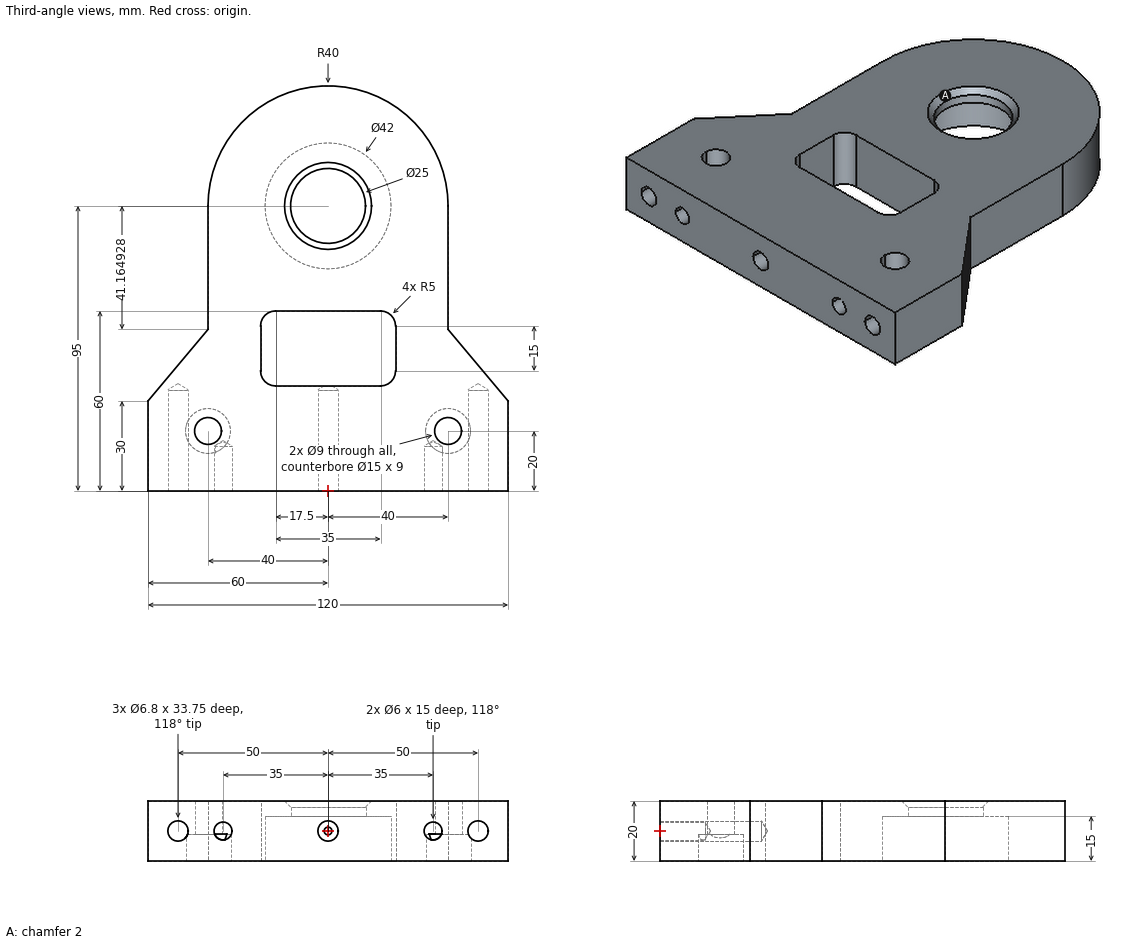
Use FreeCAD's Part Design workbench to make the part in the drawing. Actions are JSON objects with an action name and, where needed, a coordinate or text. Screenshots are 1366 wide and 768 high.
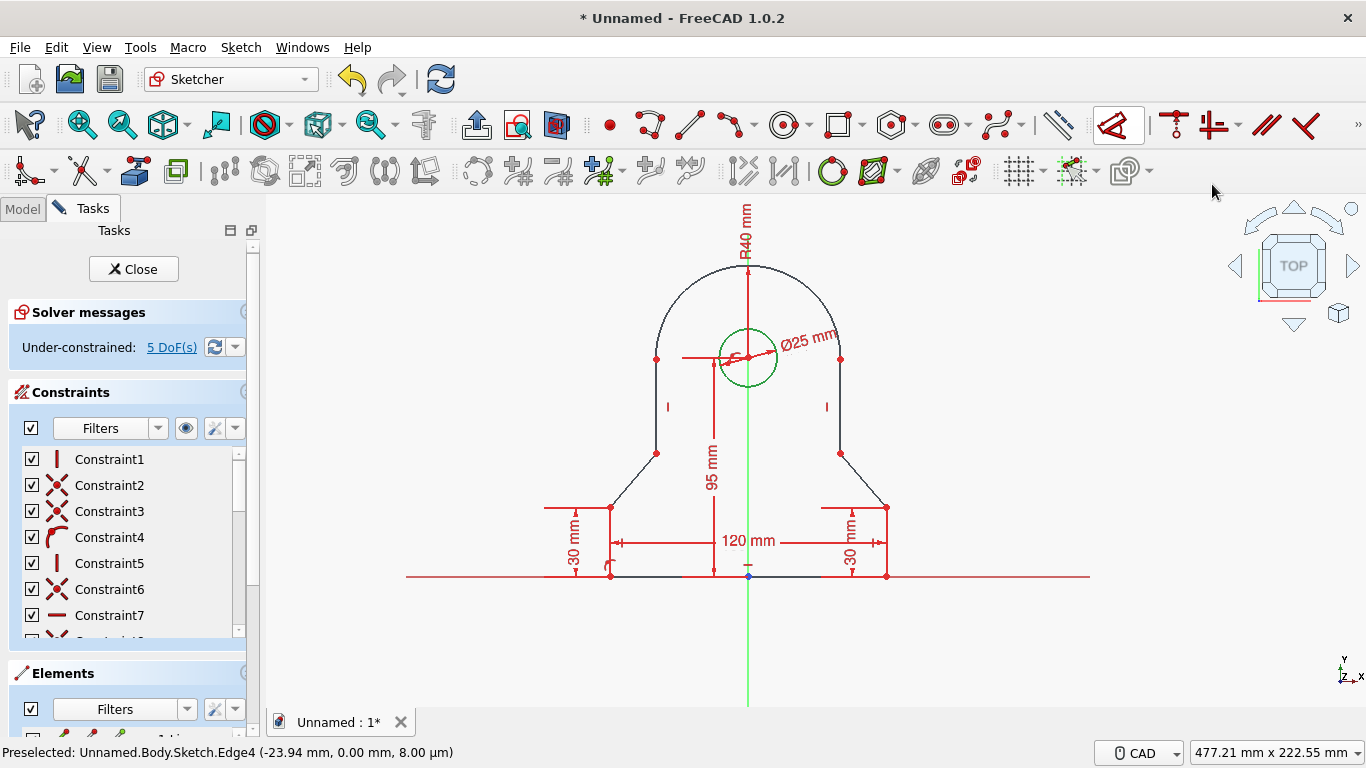
{"action": "left_click", "coordinate": [656, 359]}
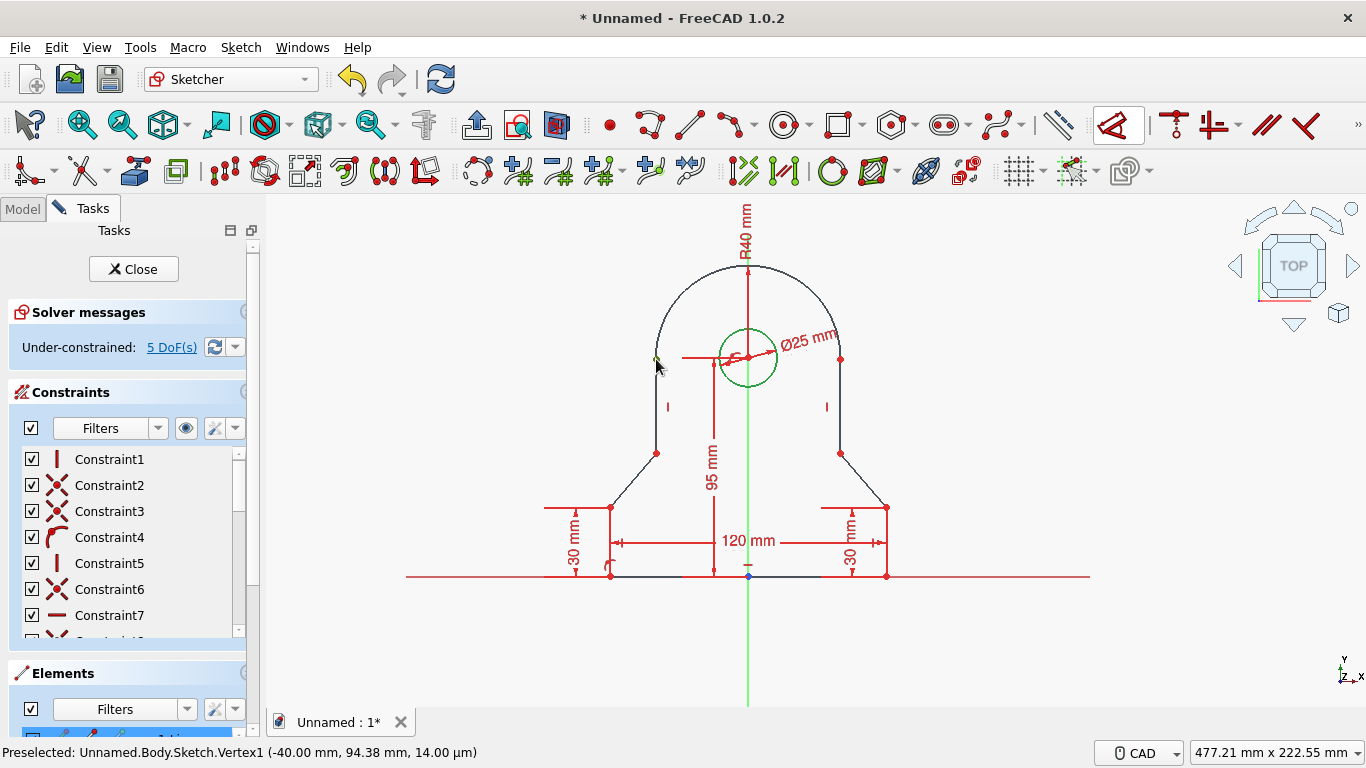
{"action": "key", "text": "i"}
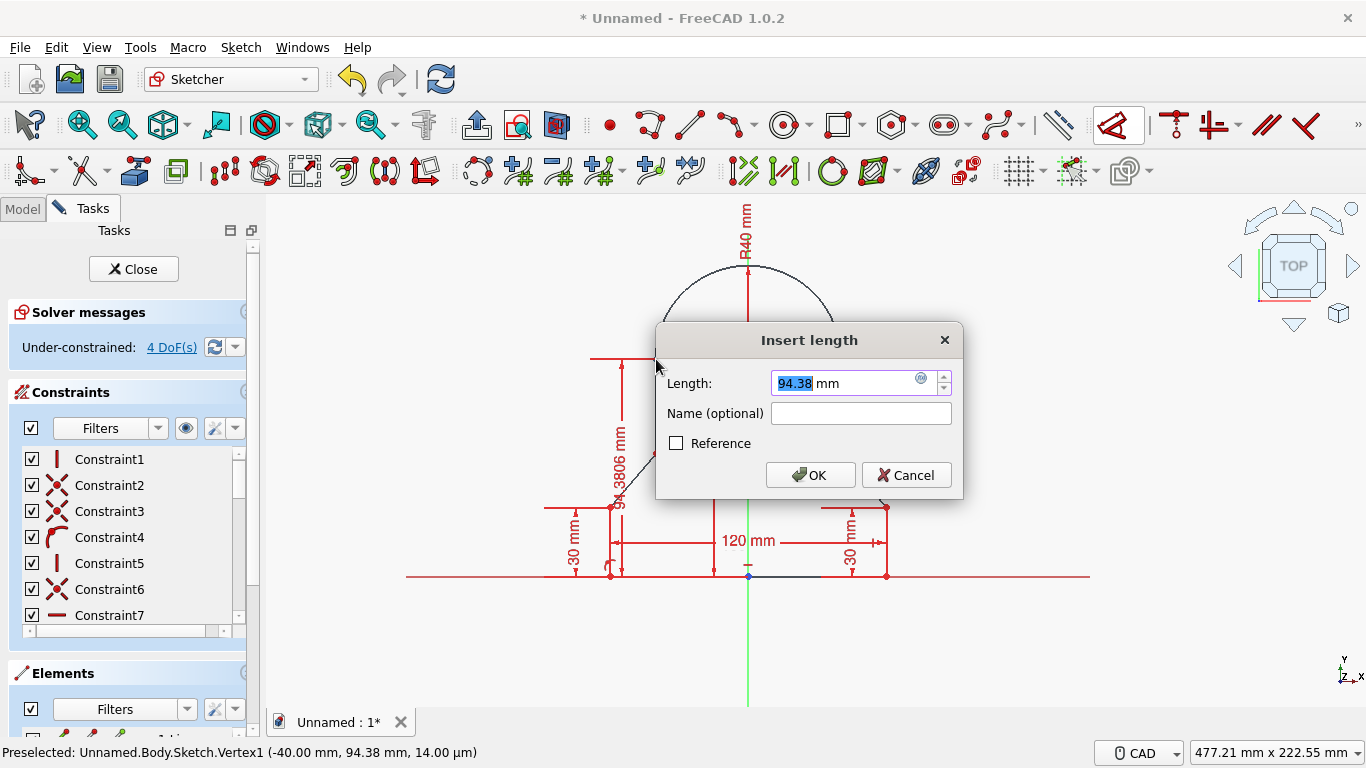
{"action": "type", "text": "95"}
{"action": "key", "text": "Return"}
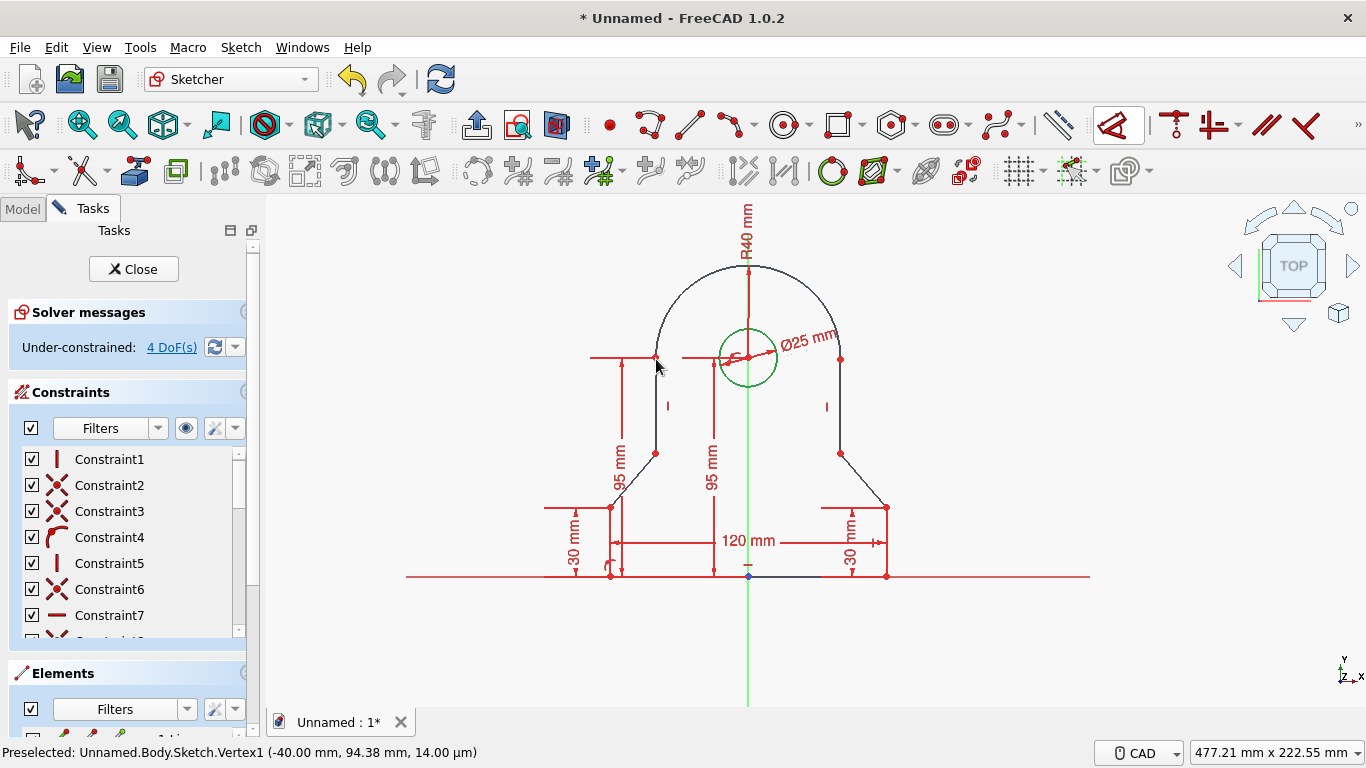
{"action": "left_click", "coordinate": [610, 508]}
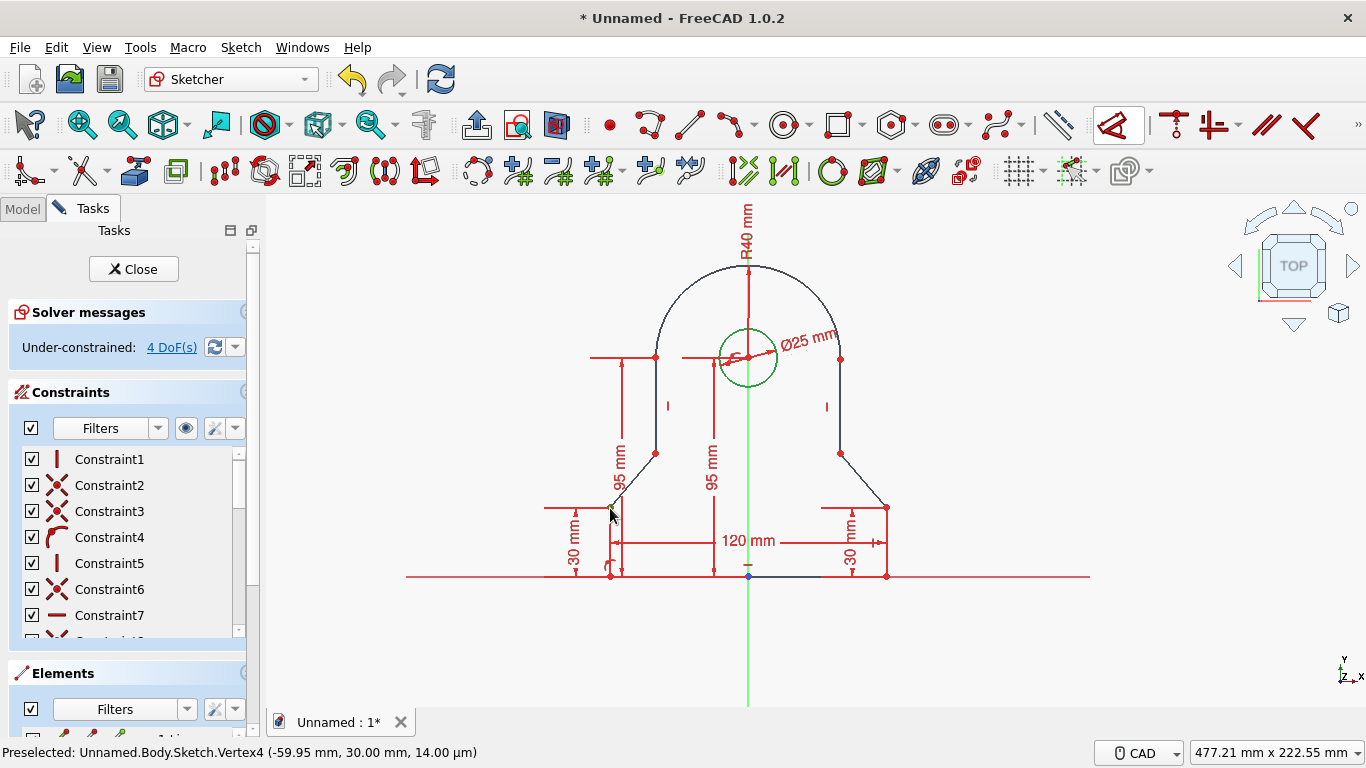
{"action": "left_click", "coordinate": [1138, 126]}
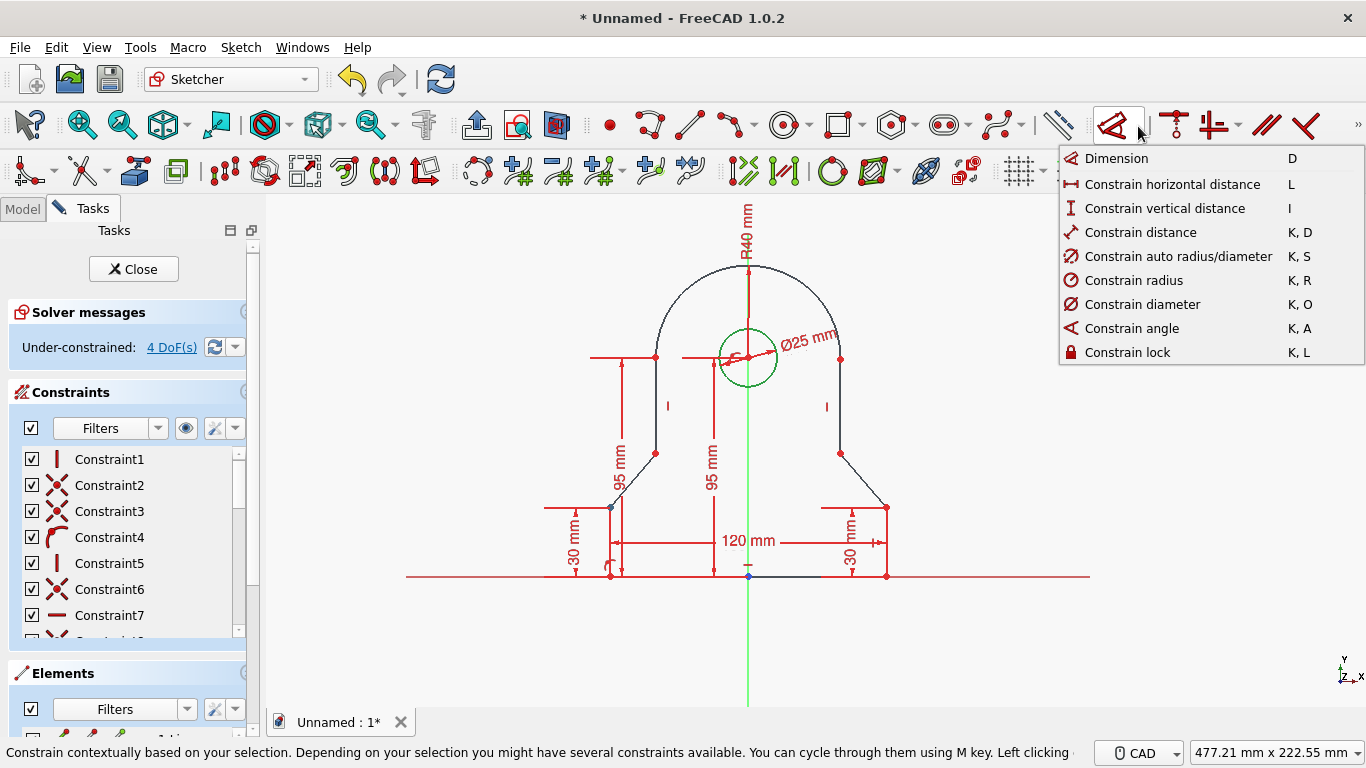
{"action": "left_click", "coordinate": [1212, 184]}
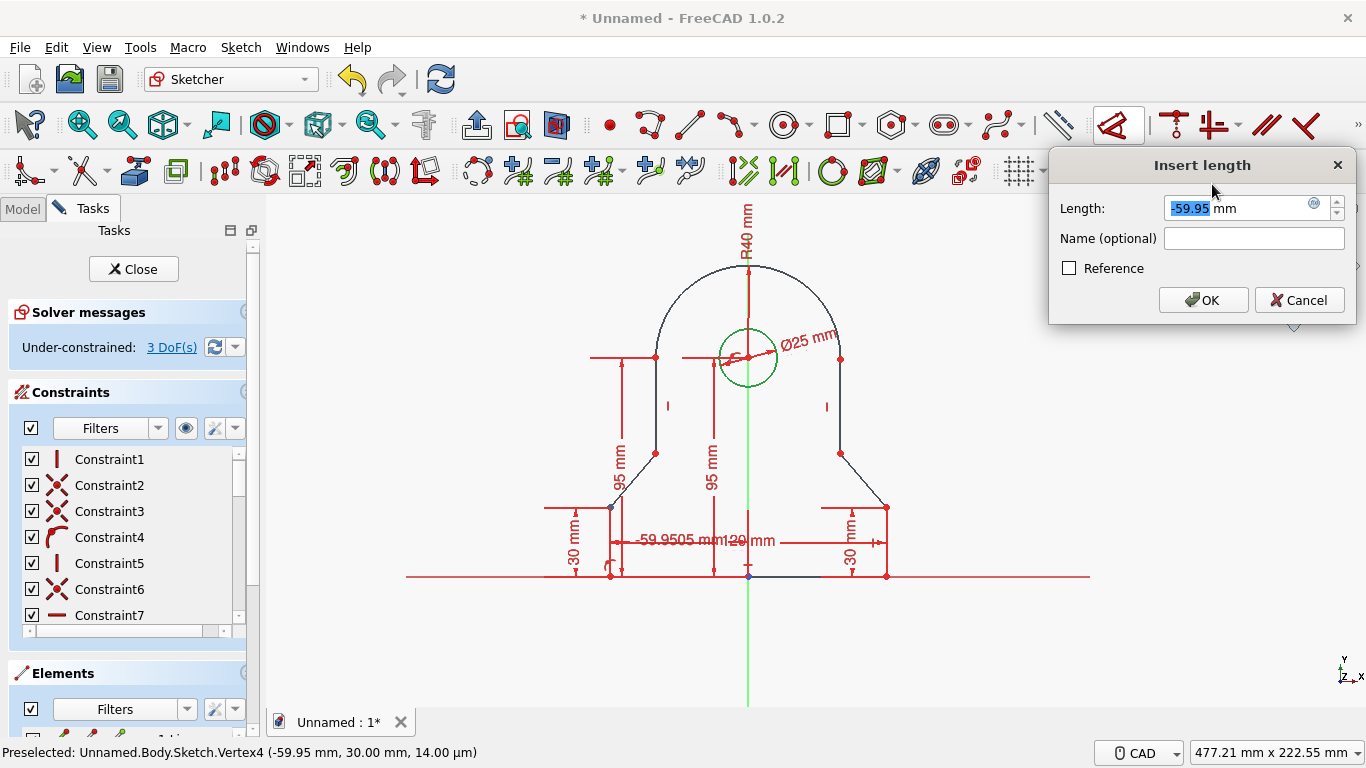
{"action": "type", "text": "-60"}
{"action": "key", "text": "Return"}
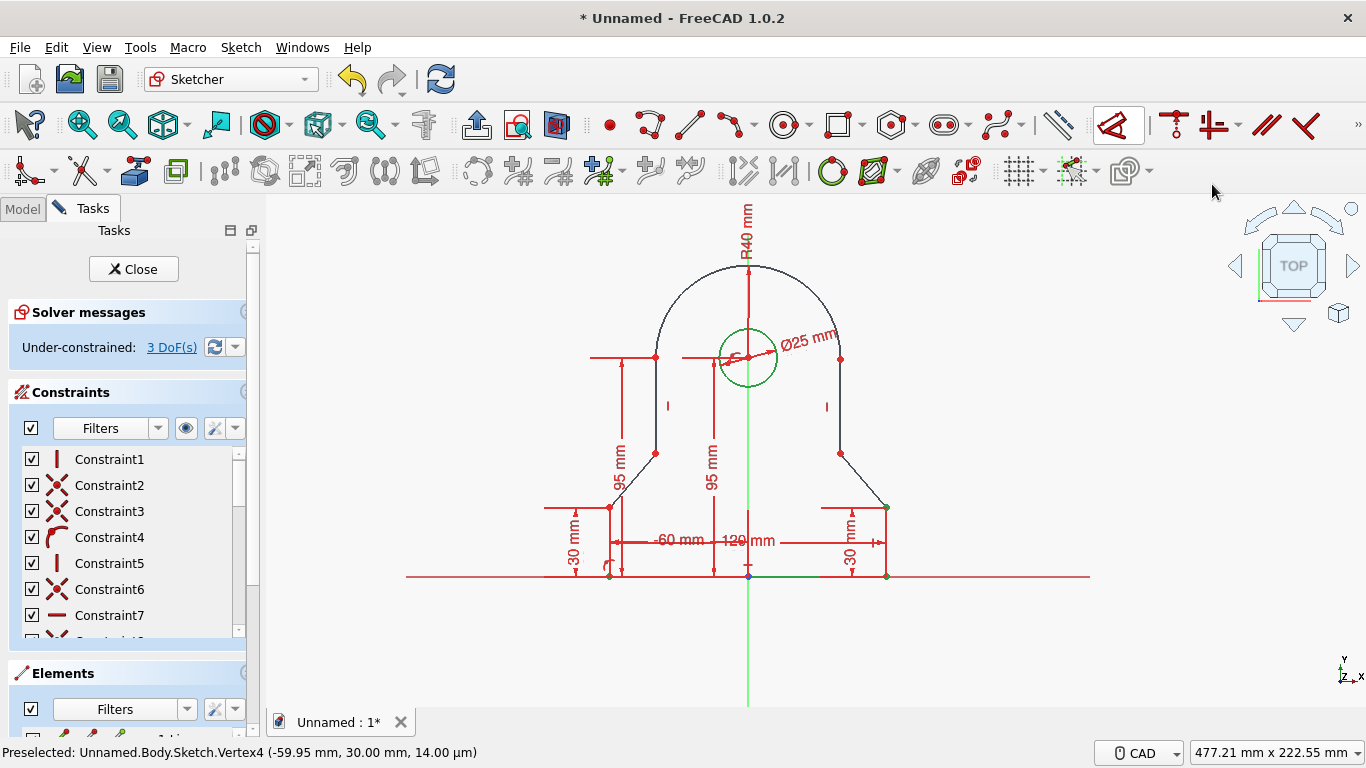
{"action": "left_click", "coordinate": [840, 359]}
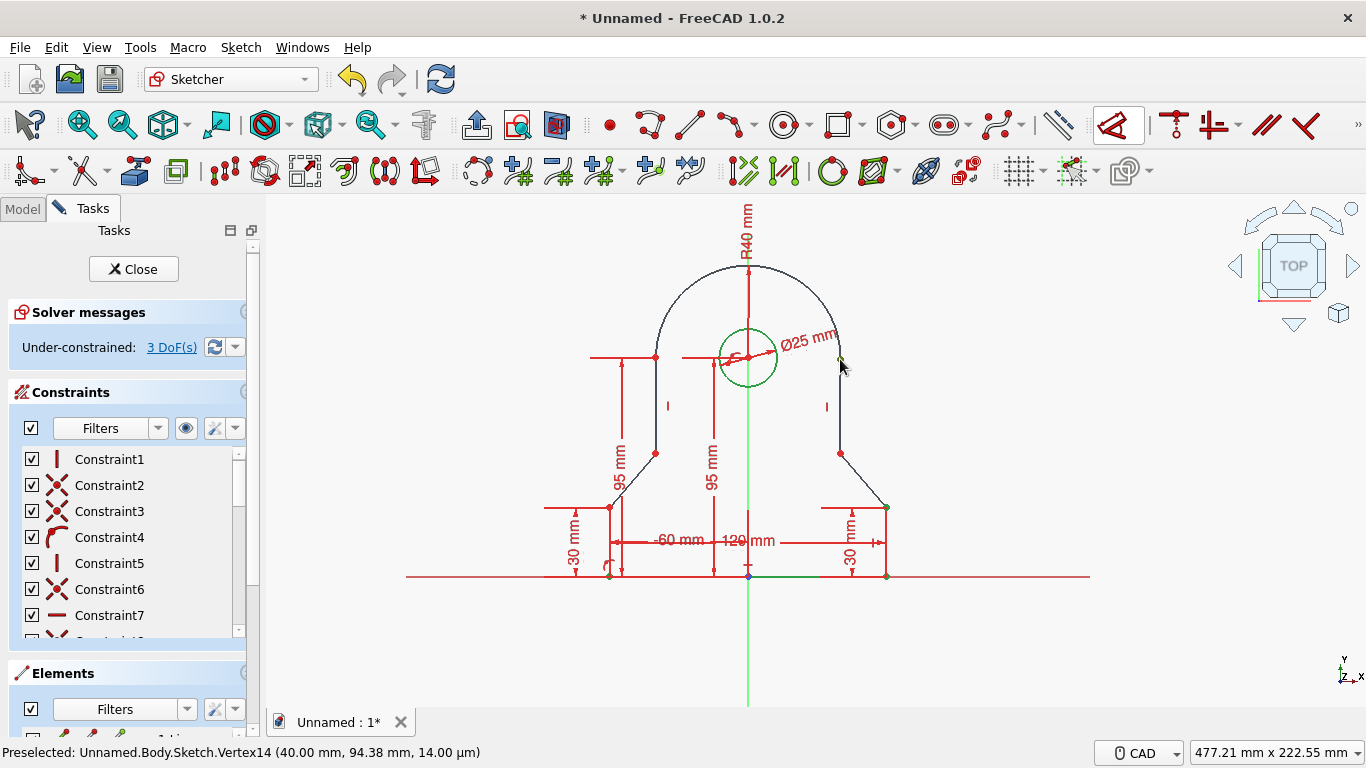
{"action": "left_click", "coordinate": [1138, 126]}